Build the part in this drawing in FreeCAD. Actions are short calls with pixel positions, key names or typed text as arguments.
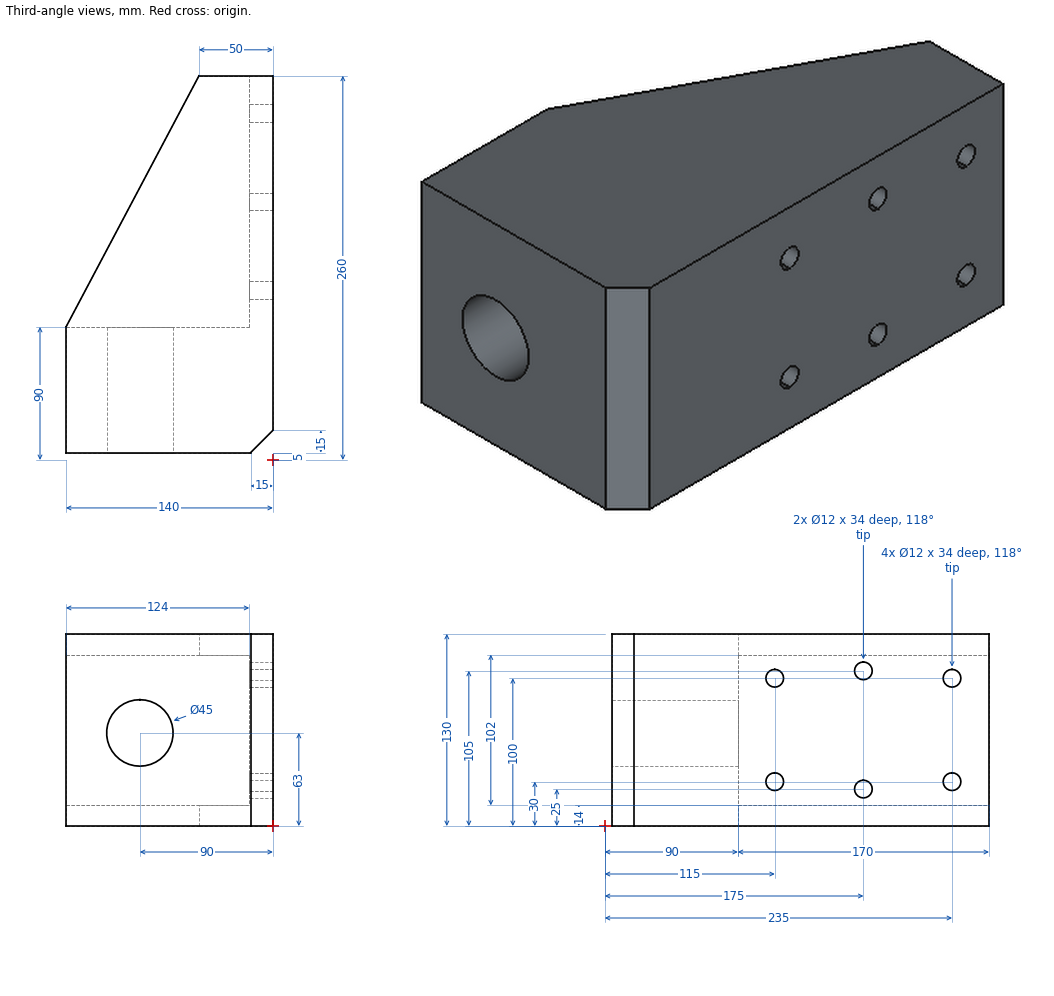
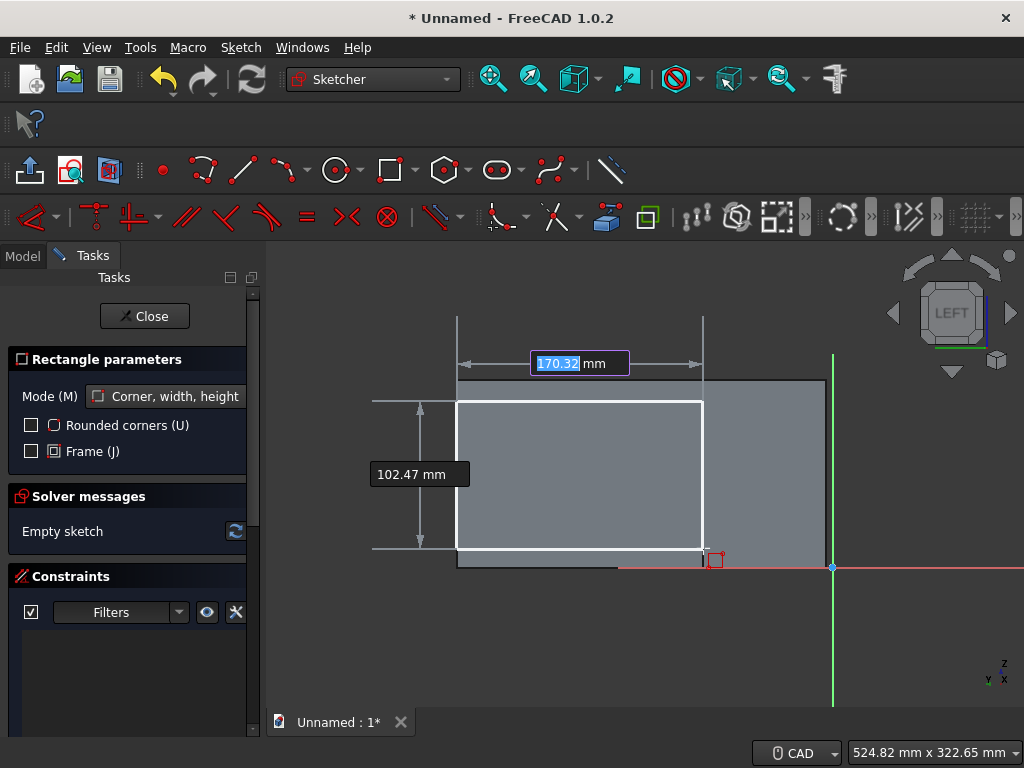
text(170)
key(Tab)
text(102)
key(Return)
key(Escape)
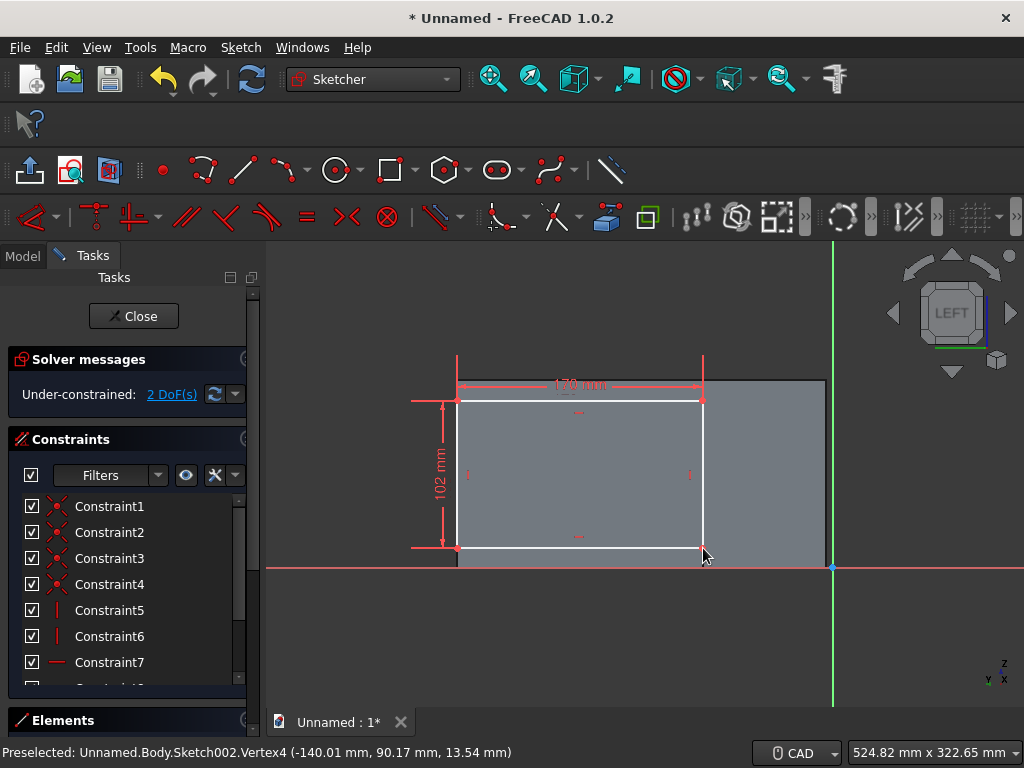
click(32, 218)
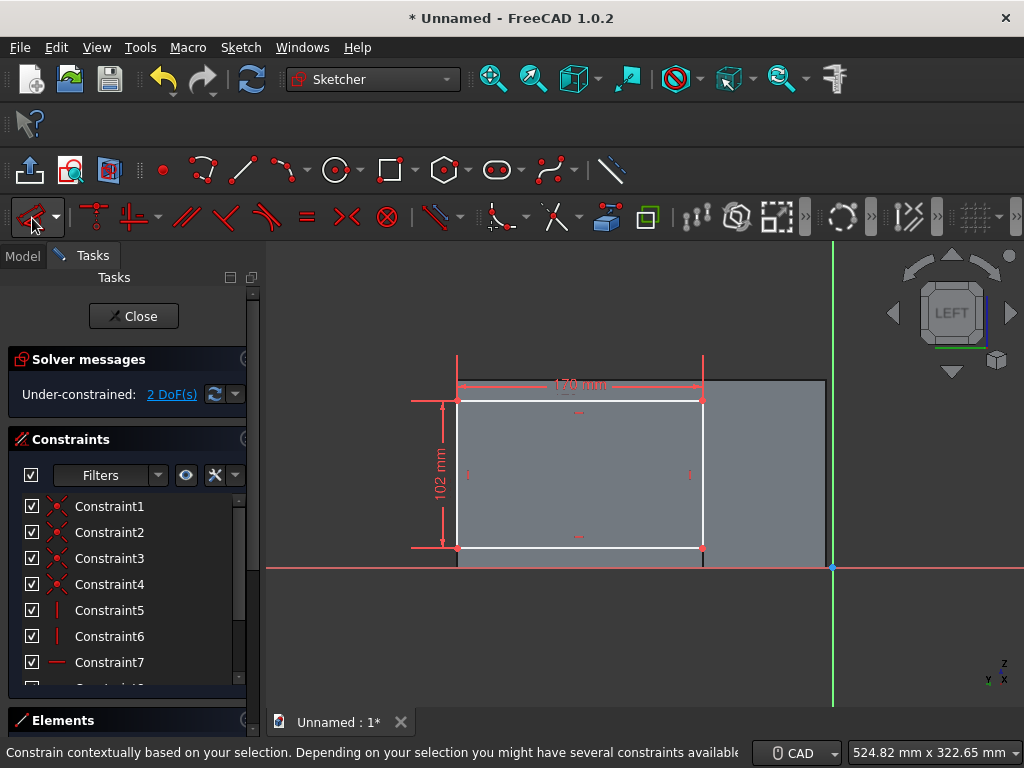
scroll(457, 548, up, 4)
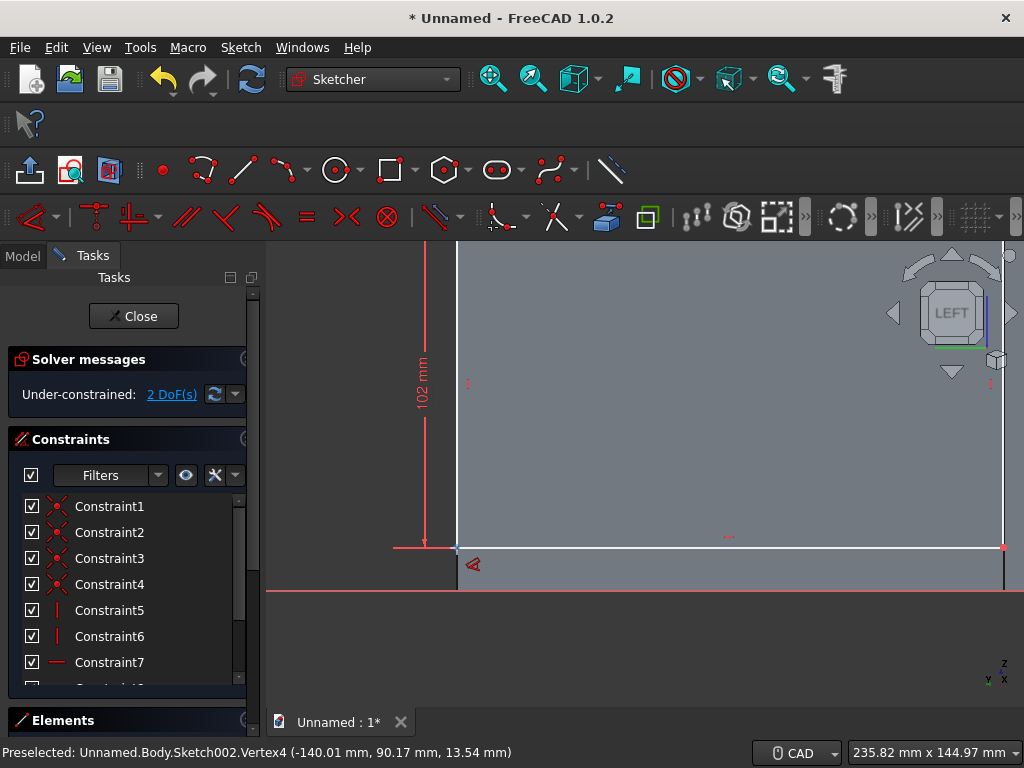
click(457, 548)
click(423, 570)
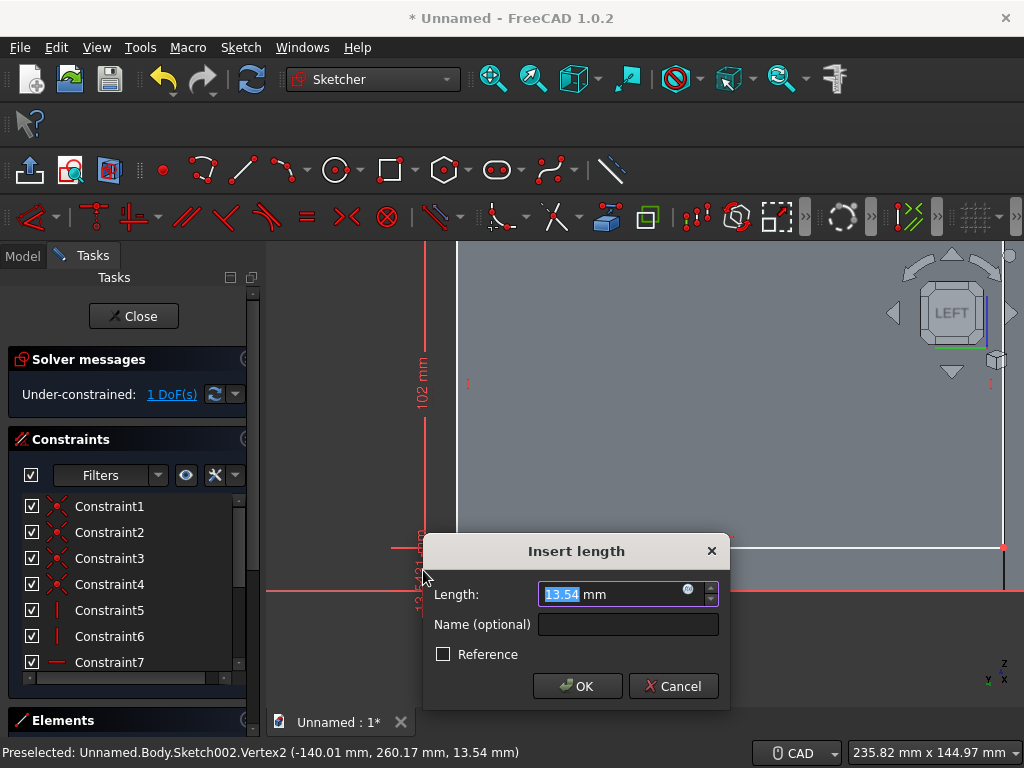
text(14)
key(Return)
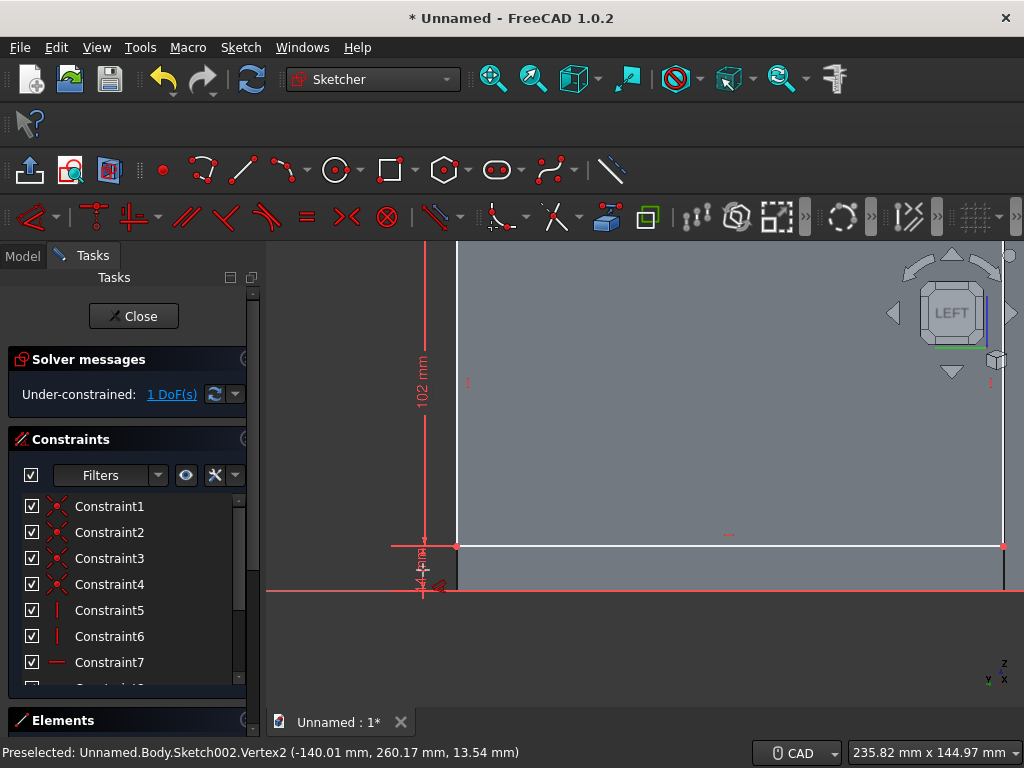
scroll(333, 530, down, 4)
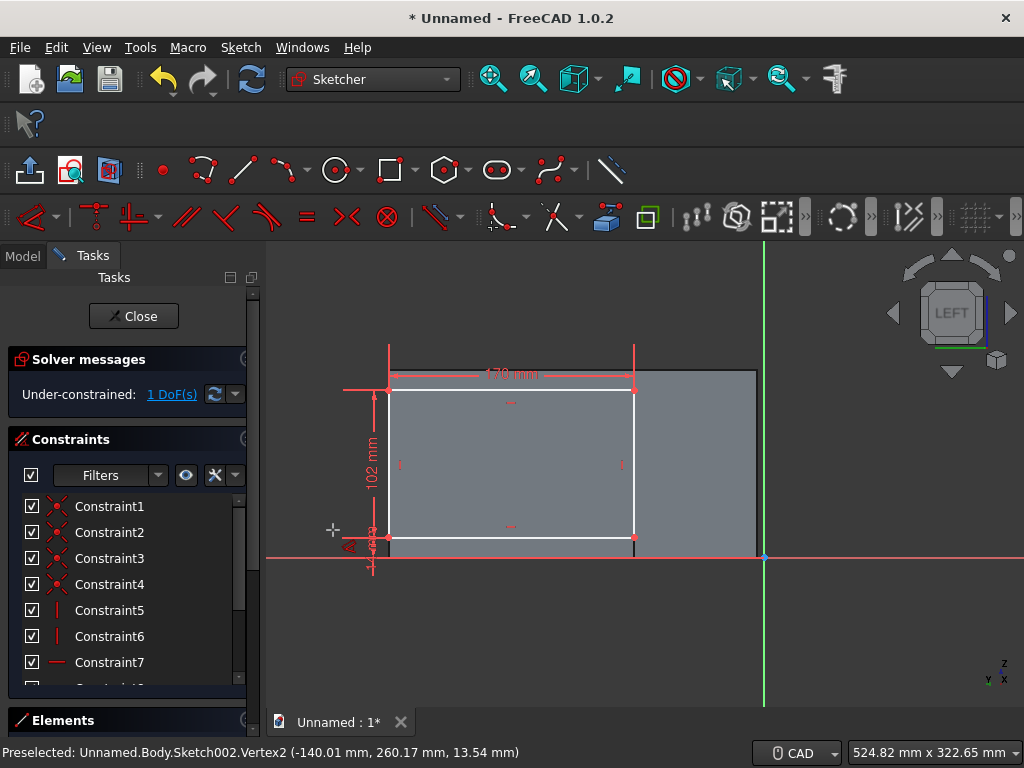
click(634, 538)
click(699, 592)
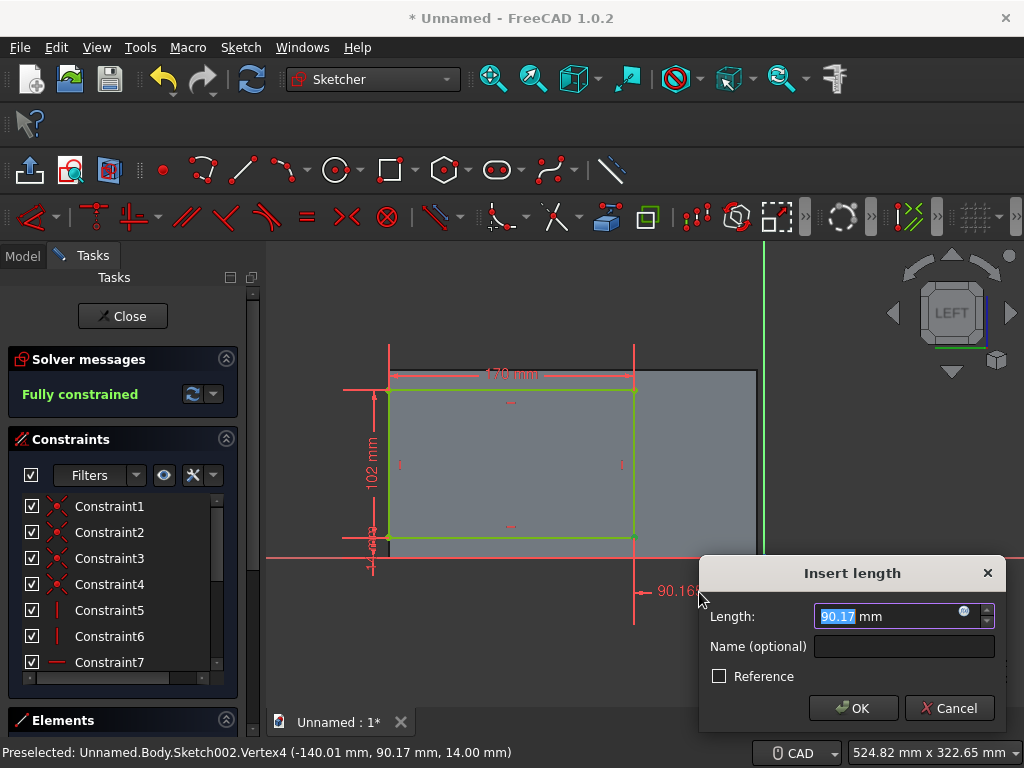
text(90)
key(Return)
key(Escape)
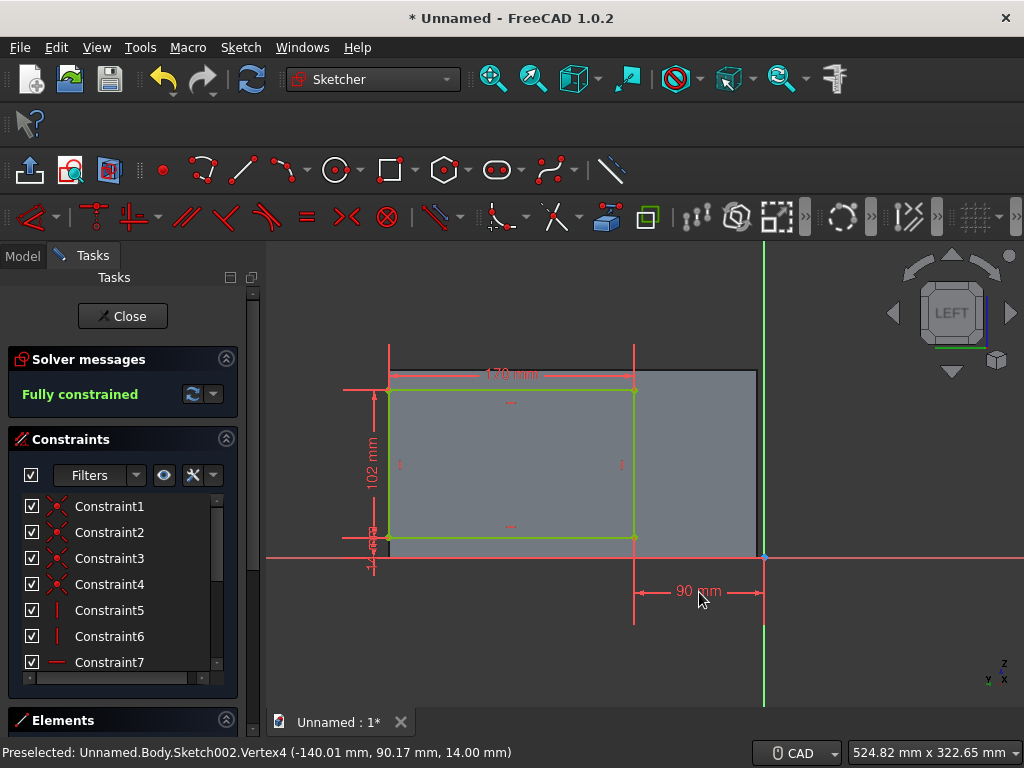
click(123, 316)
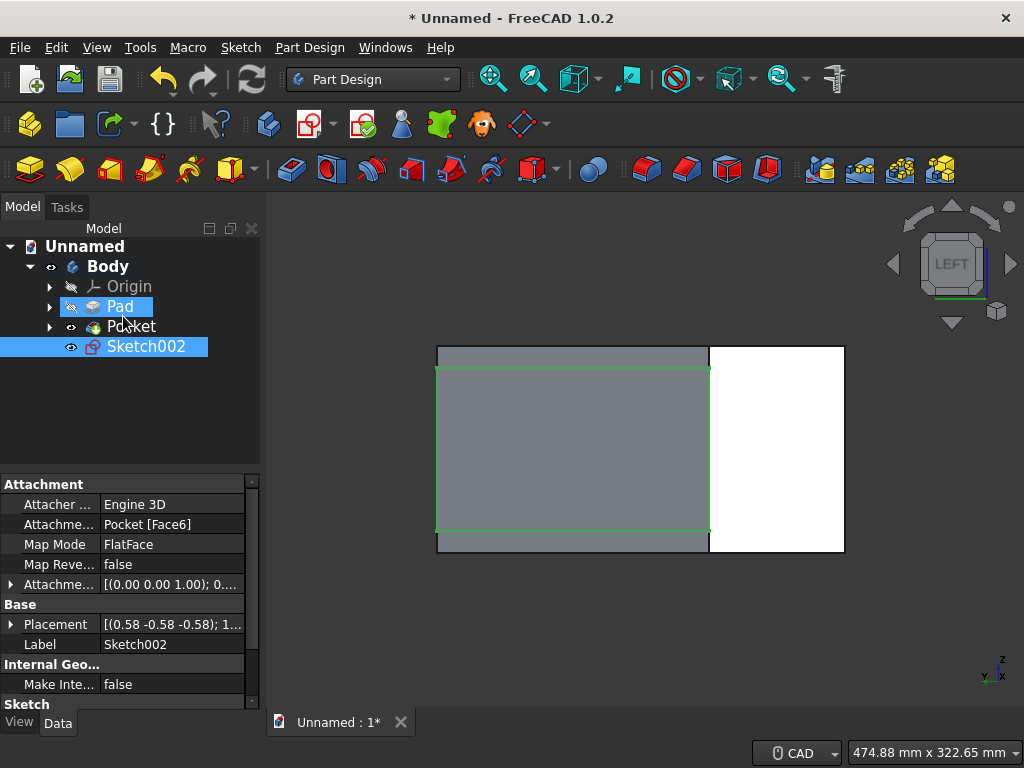
click(292, 170)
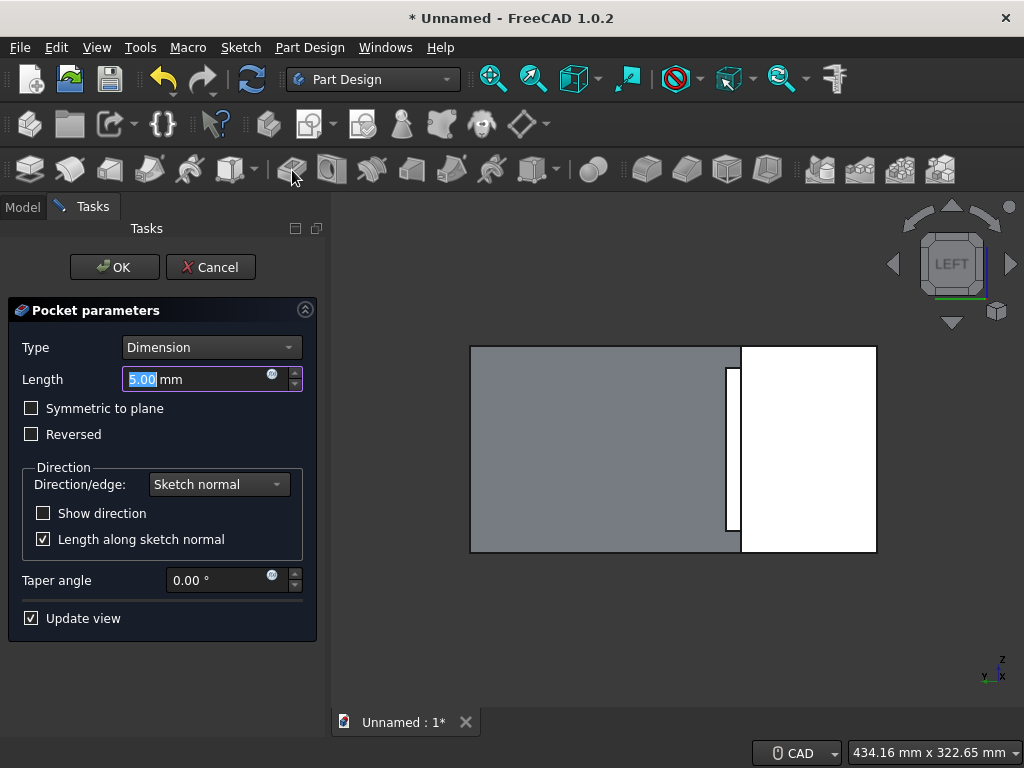
text(124)
key(Tab)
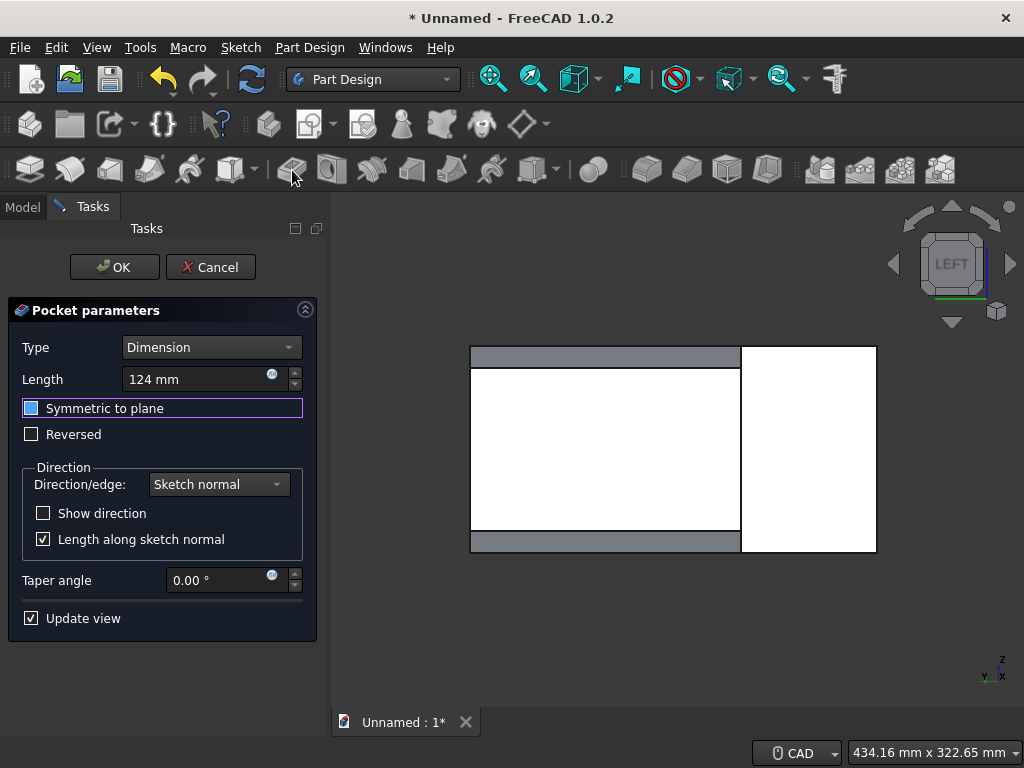
click(115, 267)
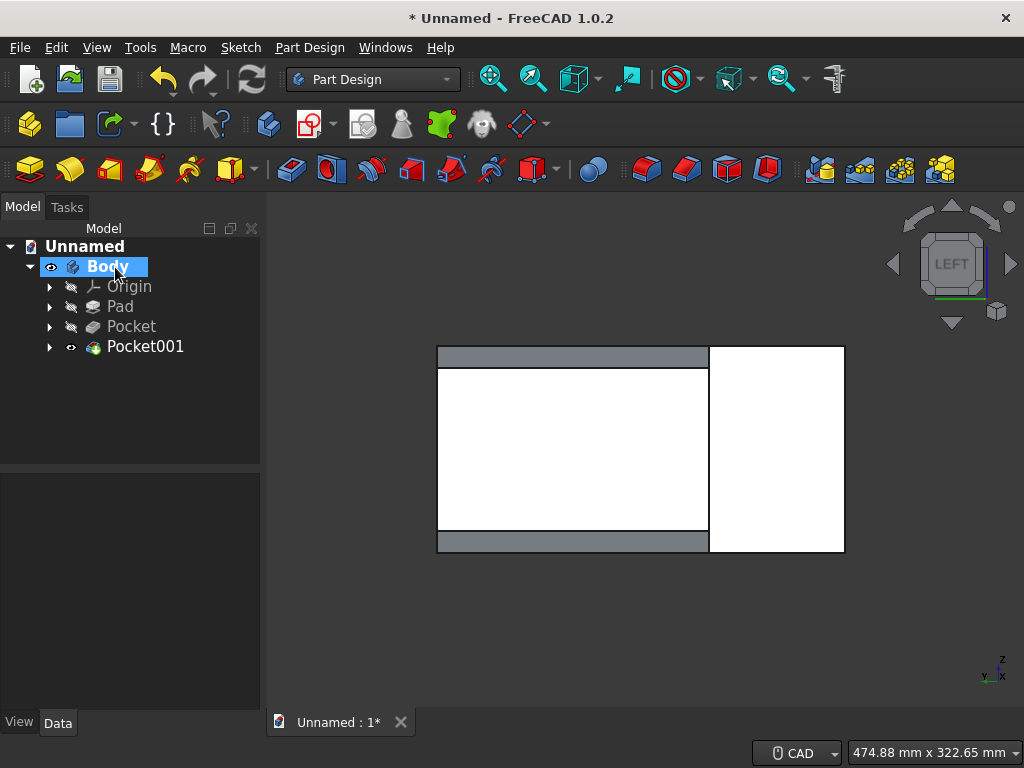
key(0)